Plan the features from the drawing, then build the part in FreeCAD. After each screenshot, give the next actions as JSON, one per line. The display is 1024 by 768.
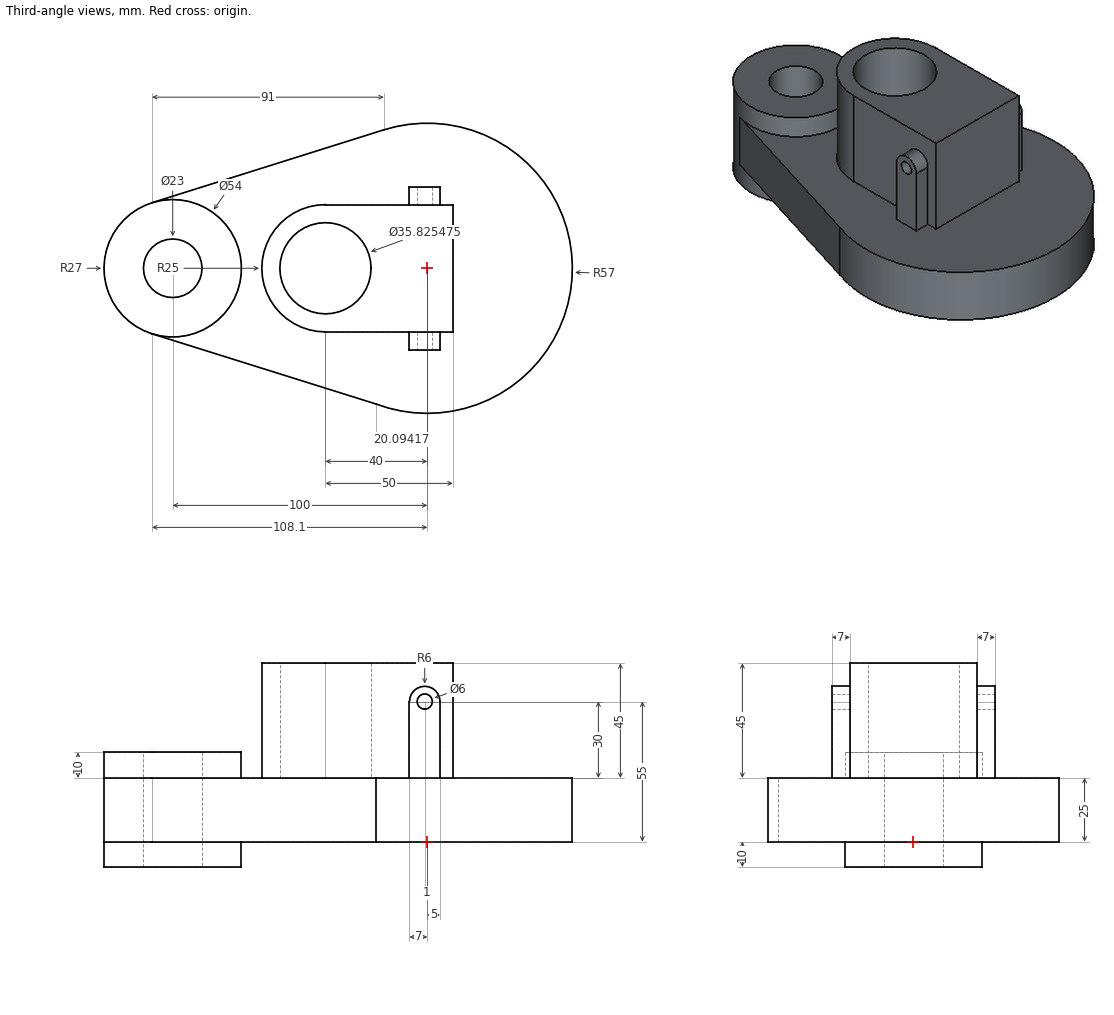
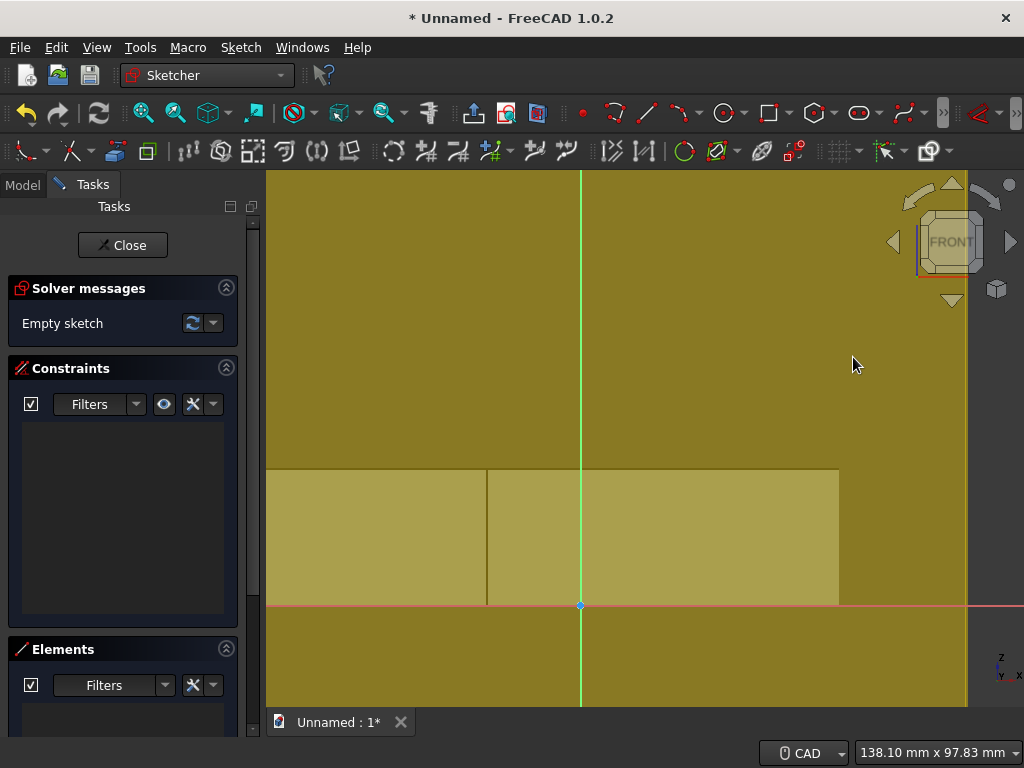
{"action": "key", "text": "g m"}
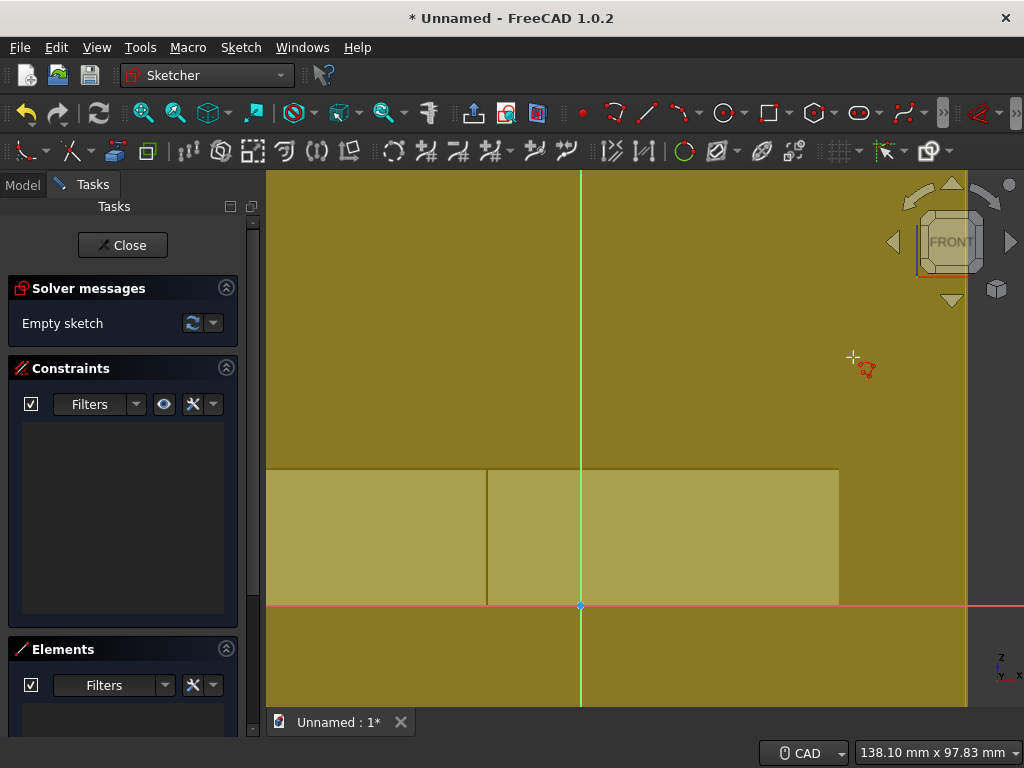
{"action": "left_click", "coordinate": [608, 304]}
{"action": "left_click", "coordinate": [608, 469]}
{"action": "left_click", "coordinate": [542, 469]}
{"action": "left_click", "coordinate": [542, 304]}
{"action": "right_click", "coordinate": [542, 304]}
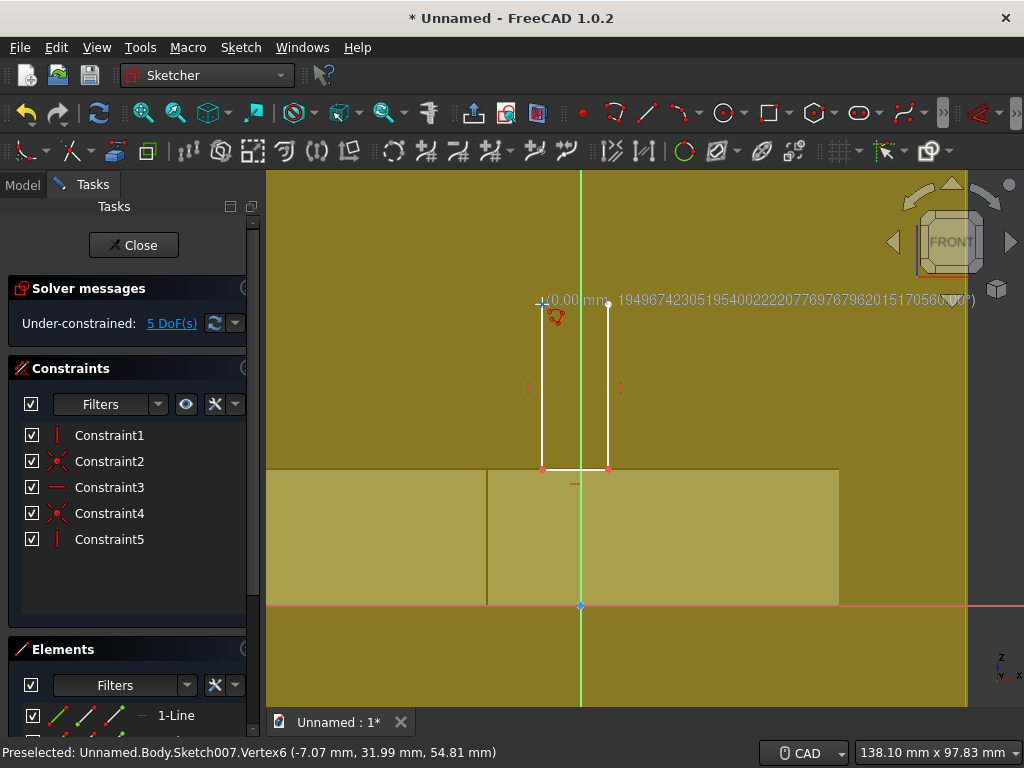
{"action": "key", "text": "g 3 a"}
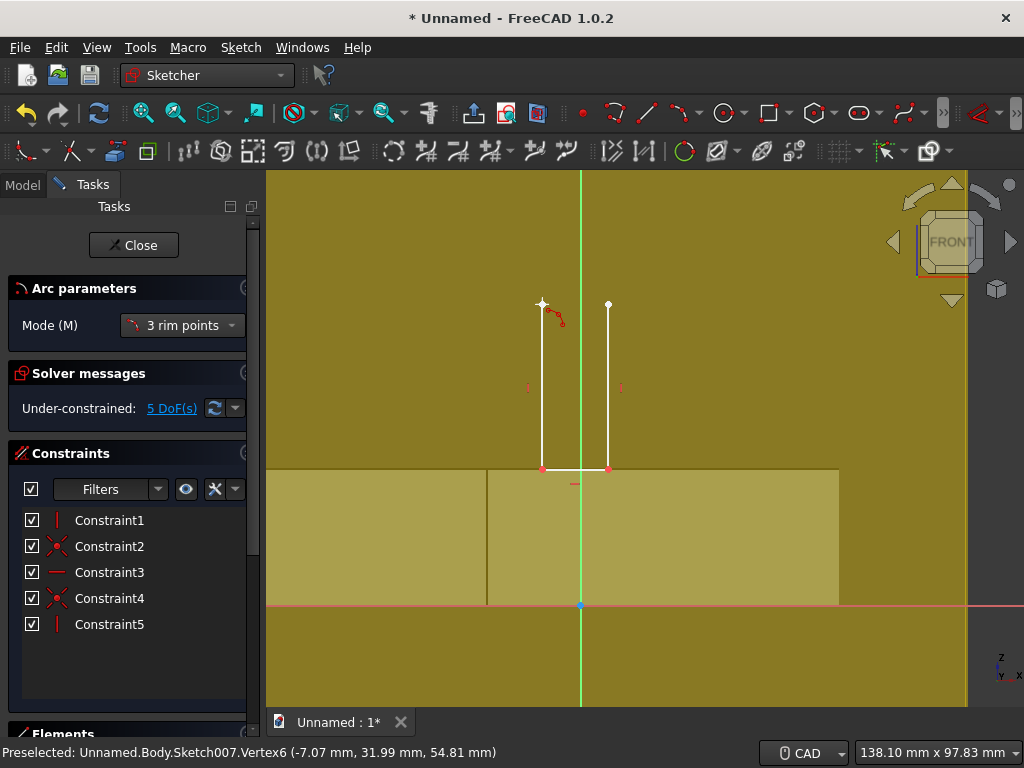
{"action": "left_click", "coordinate": [542, 305]}
{"action": "left_click", "coordinate": [608, 305]}
{"action": "left_click", "coordinate": [565, 273]}
{"action": "key", "text": "Escape"}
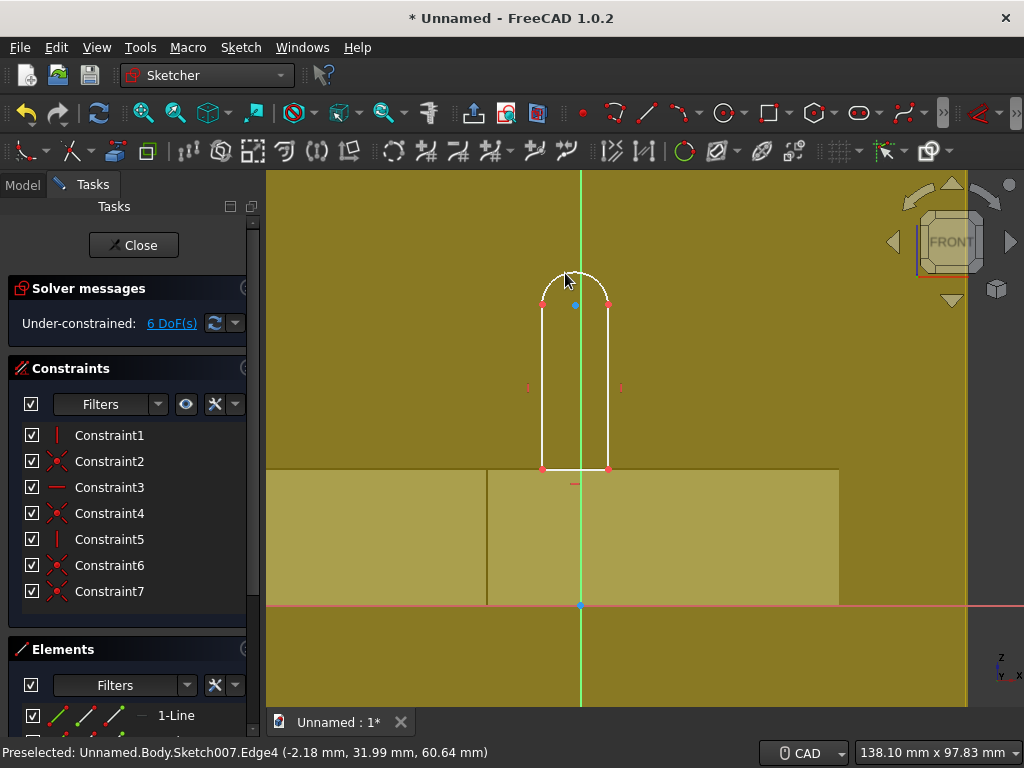
{"action": "left_click", "coordinate": [608, 355]}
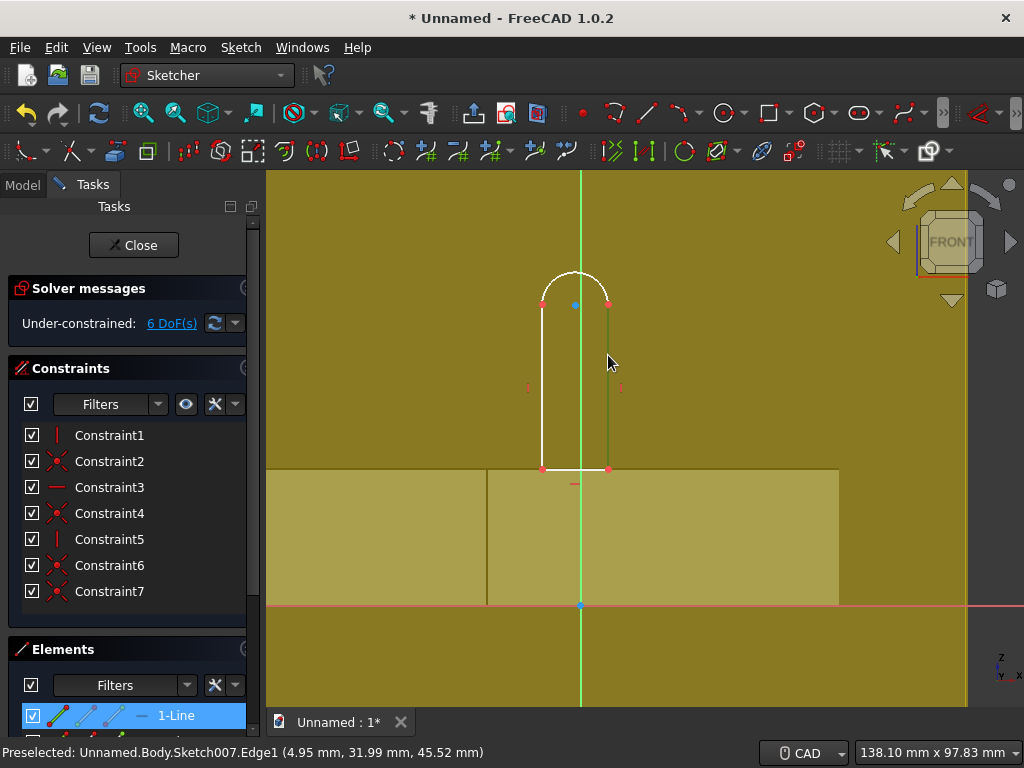
{"action": "left_click", "coordinate": [594, 279]}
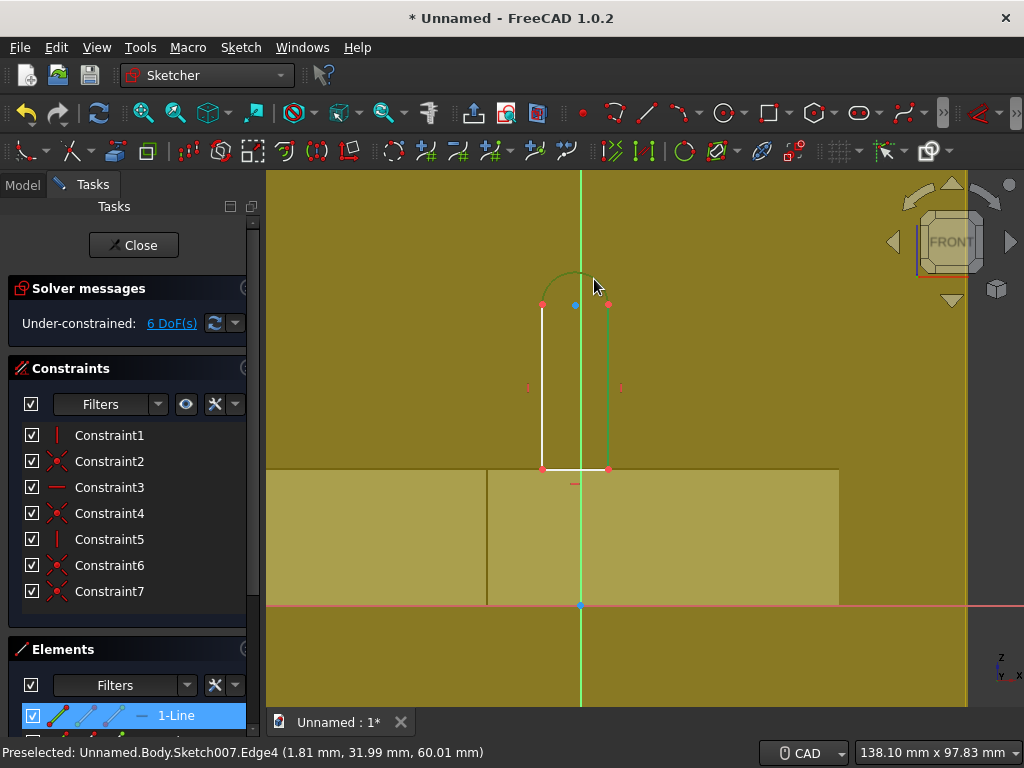
{"action": "key", "text": "t"}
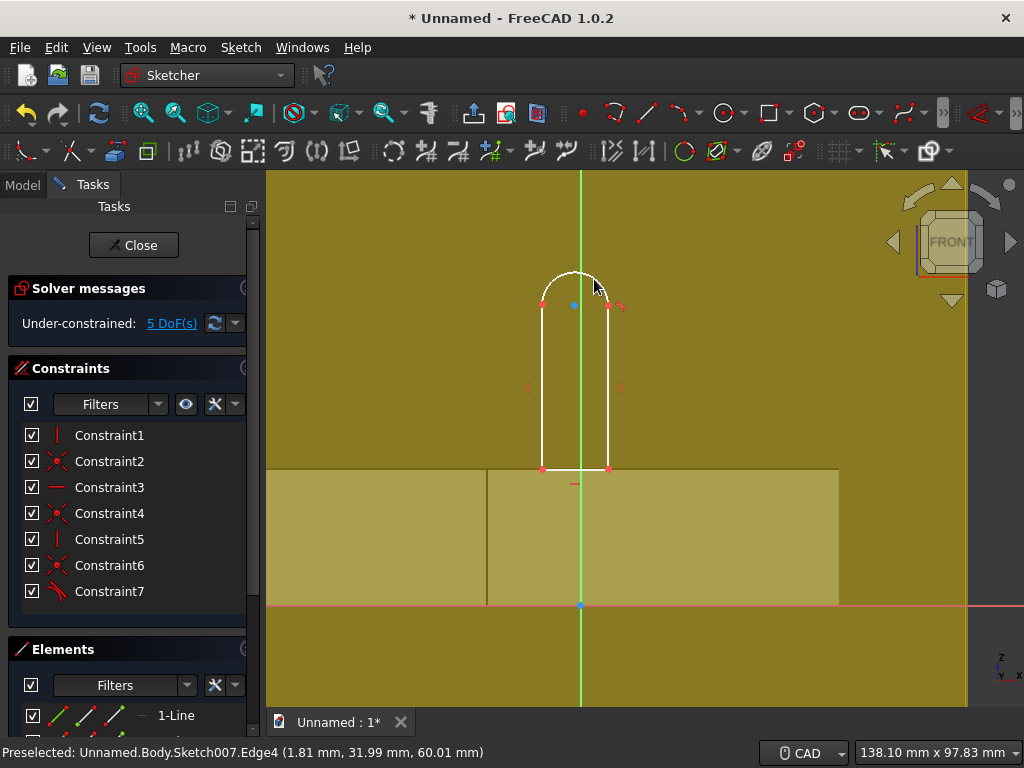
{"action": "left_click", "coordinate": [542, 421]}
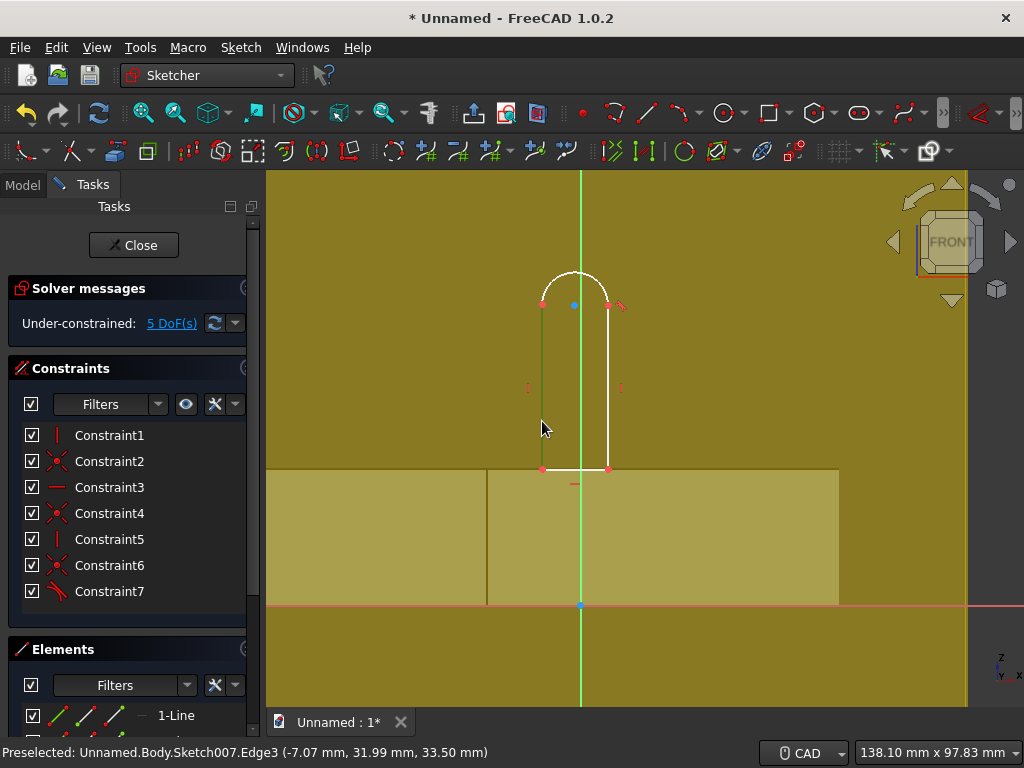
{"action": "left_click", "coordinate": [595, 279]}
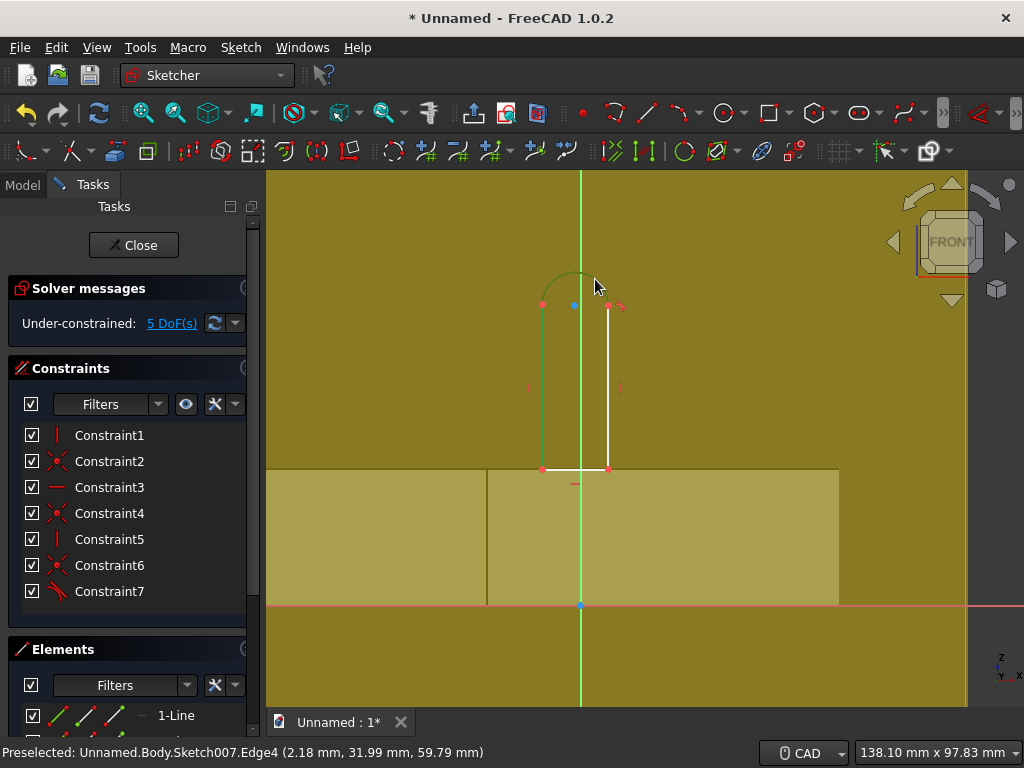
{"action": "key", "text": "t"}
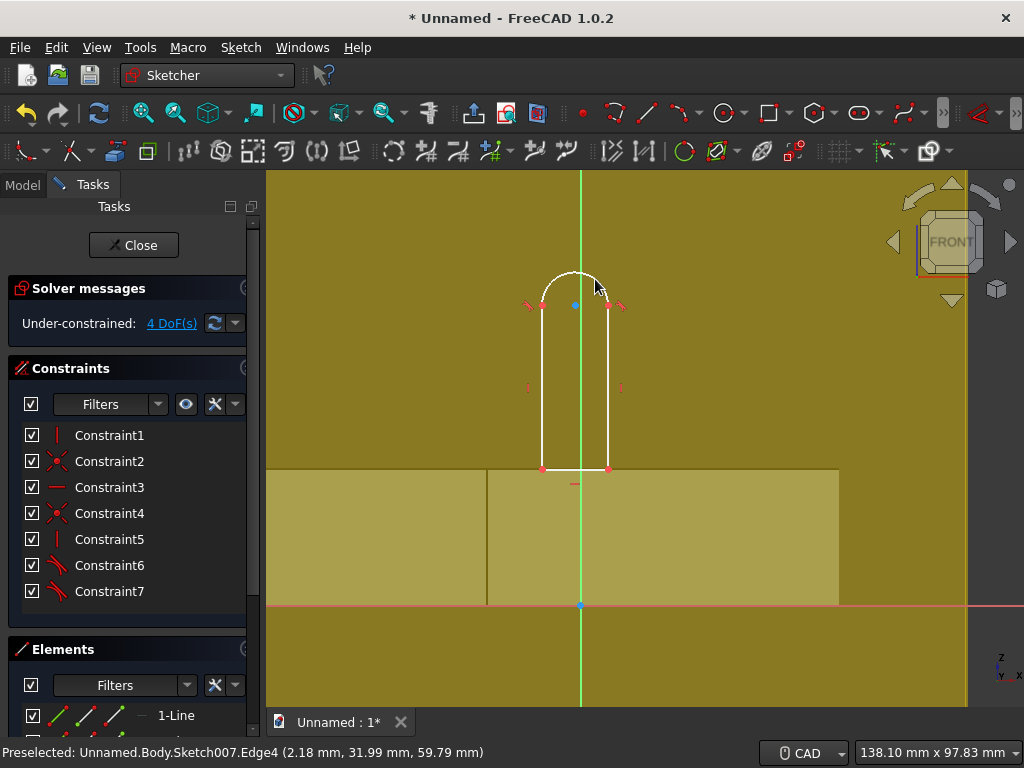
{"action": "key", "text": "d"}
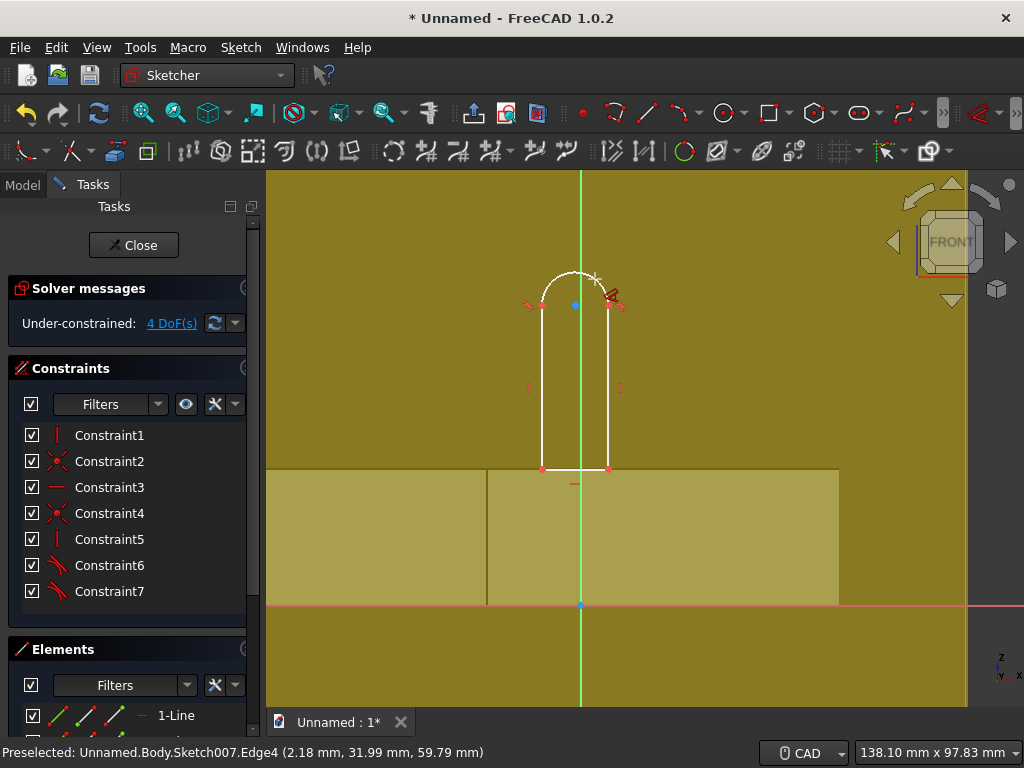
{"action": "left_click", "coordinate": [594, 279]}
{"action": "left_click", "coordinate": [613, 253]}